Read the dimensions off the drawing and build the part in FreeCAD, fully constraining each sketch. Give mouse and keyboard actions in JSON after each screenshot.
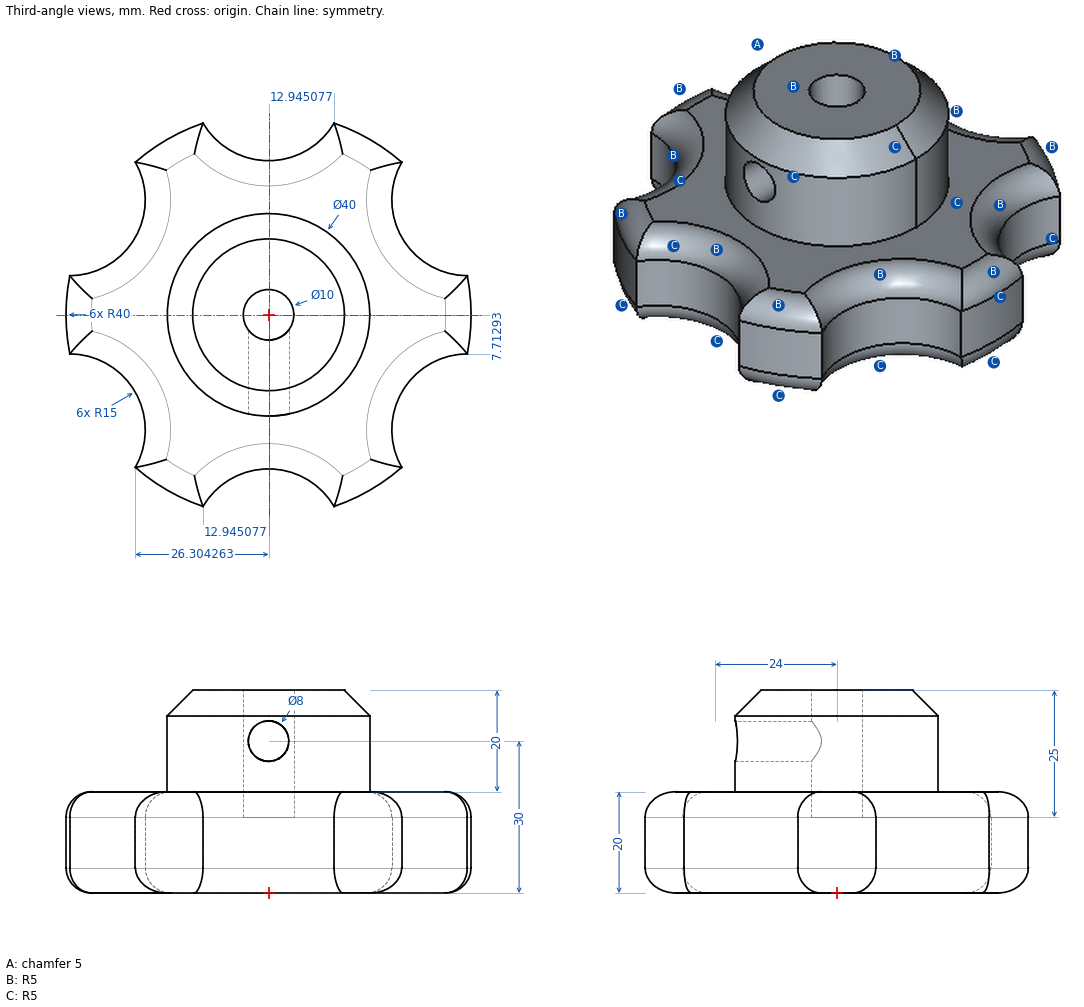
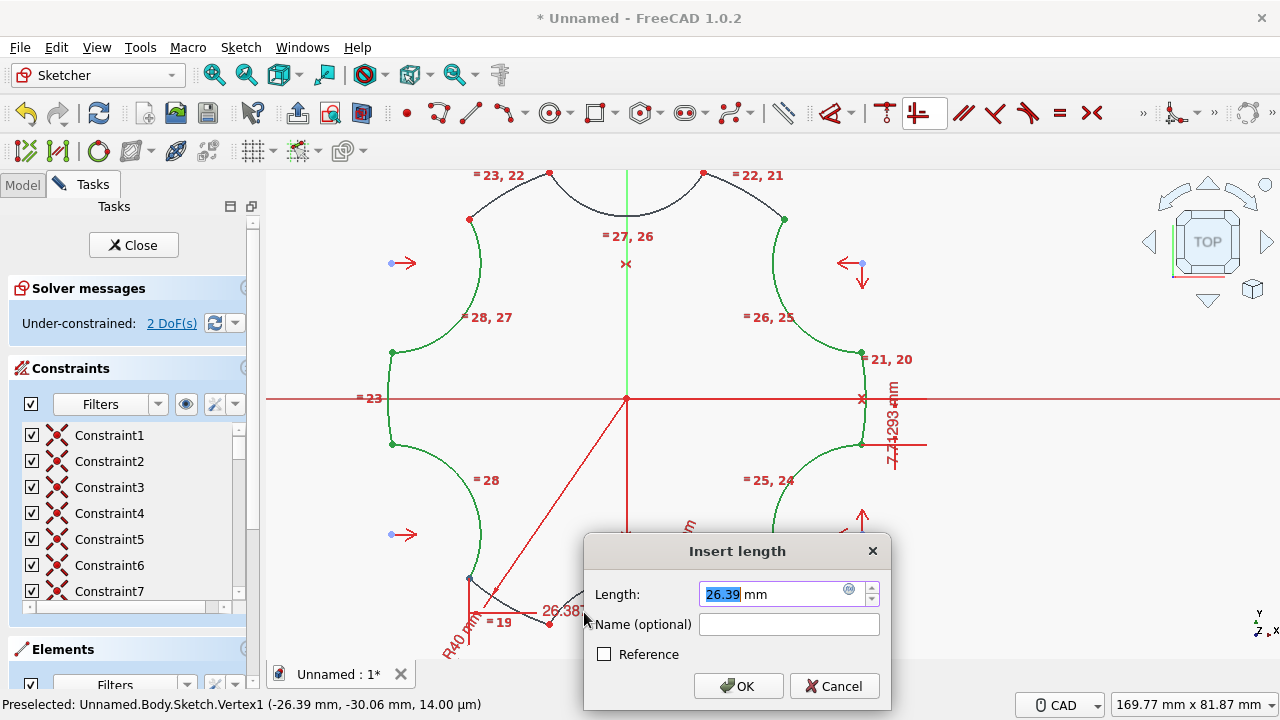
{"action": "type", "text": "26.304263"}
{"action": "key", "text": "Return"}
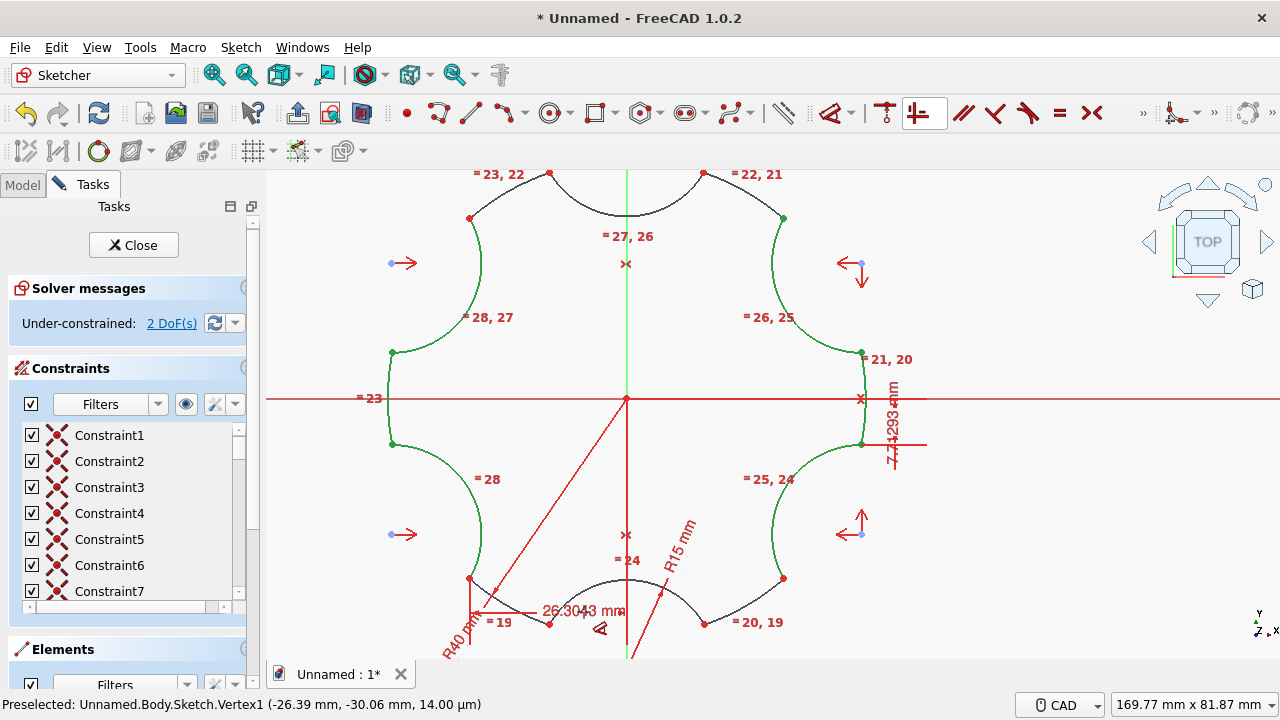
{"action": "left_click", "coordinate": [549, 625]}
{"action": "left_click", "coordinate": [588, 365]}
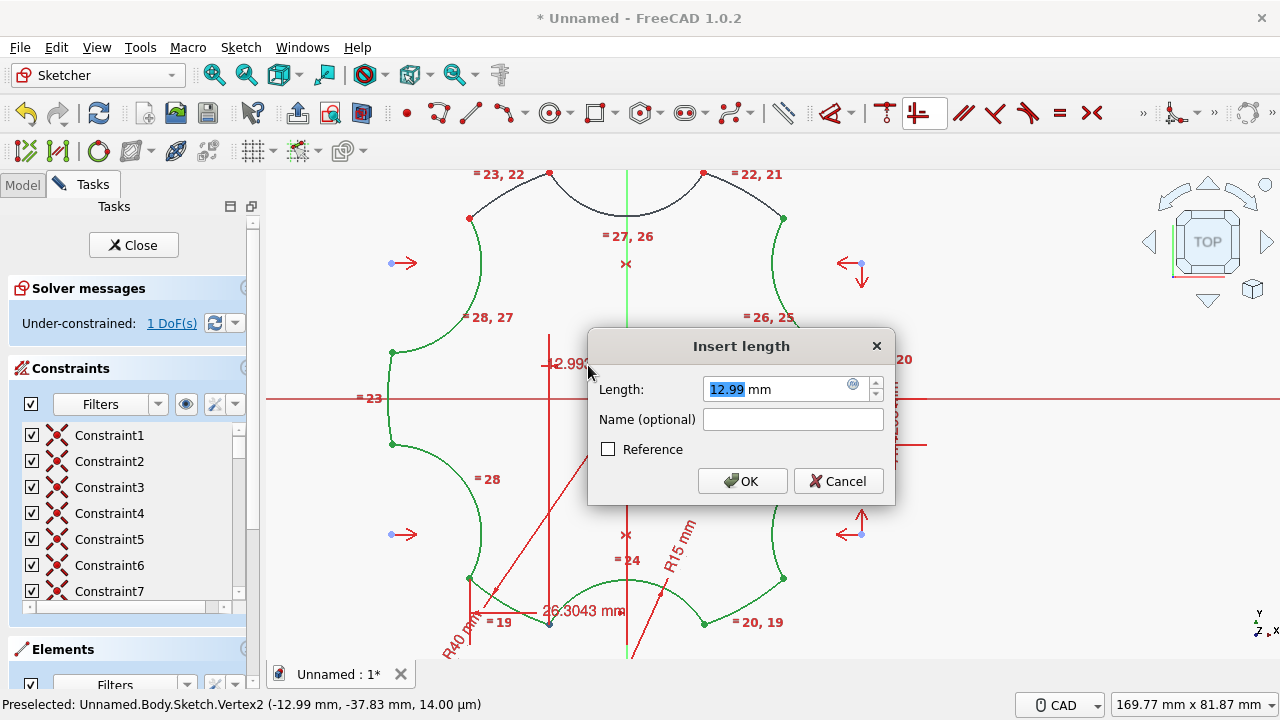
{"action": "type", "text": "12.945077"}
{"action": "key", "text": "Return"}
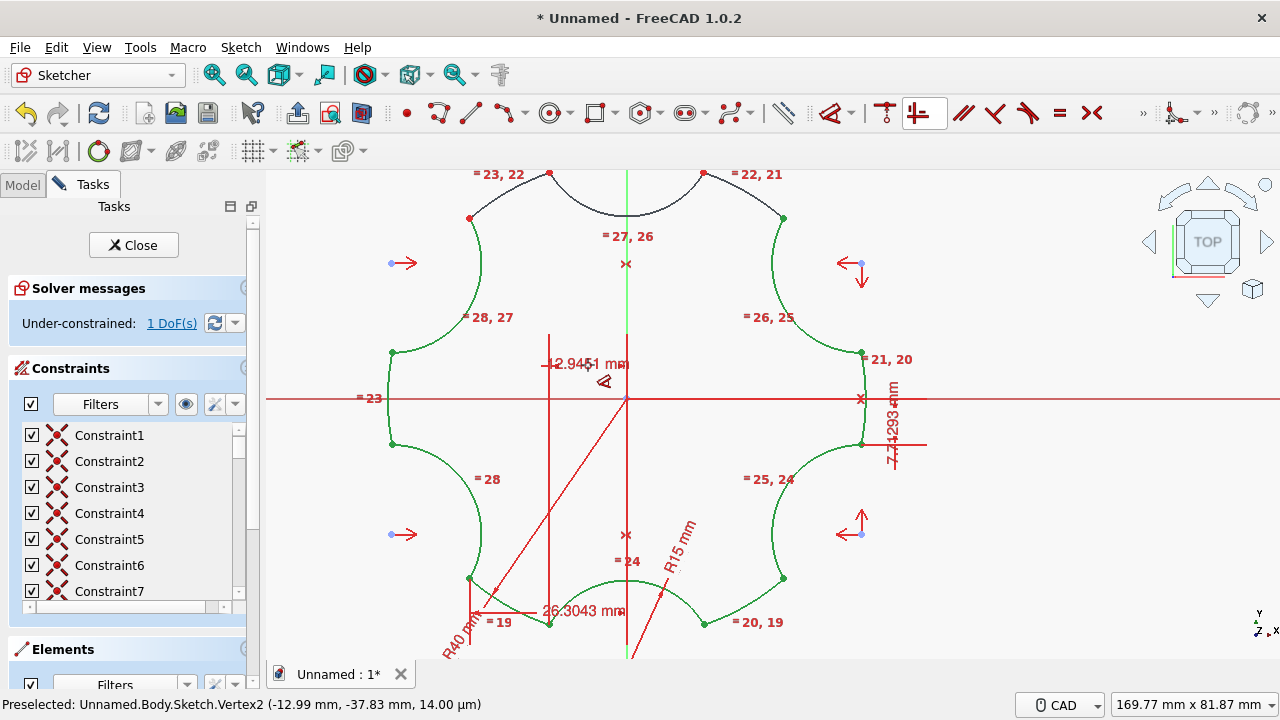
{"action": "scroll", "coordinate": [863, 446], "scroll_direction": "down", "scroll_amount": 2}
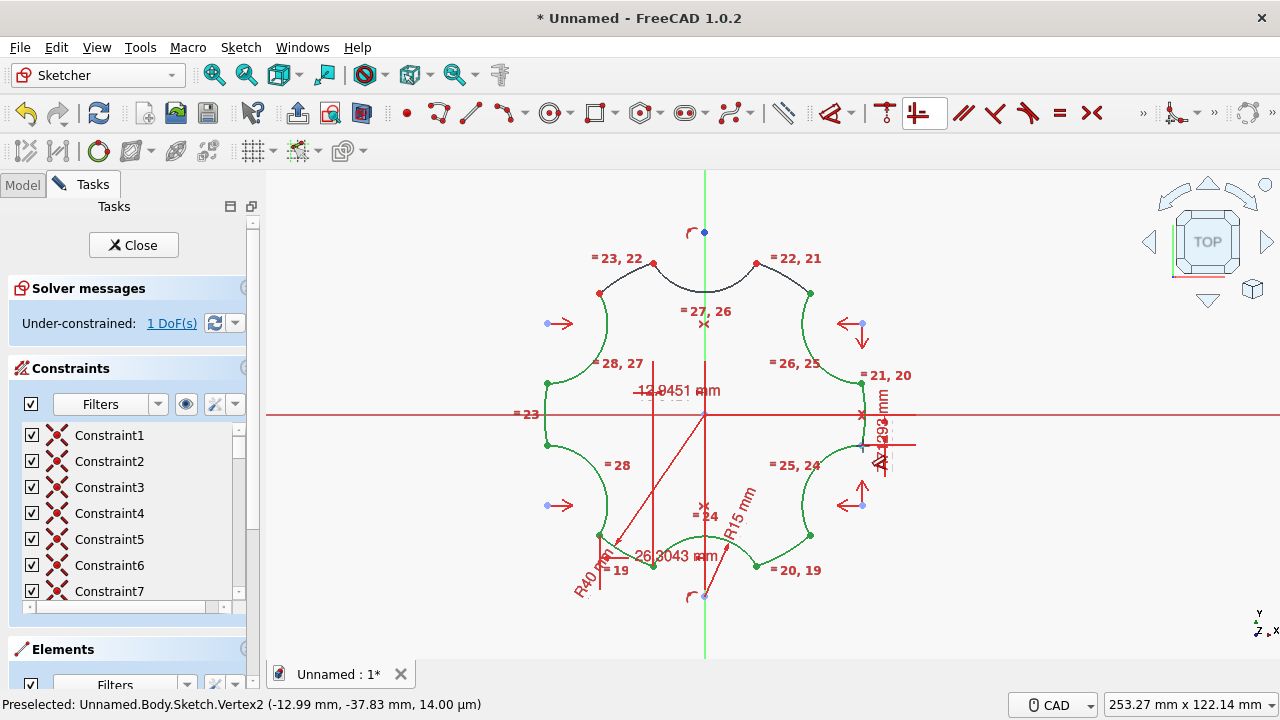
{"action": "left_click", "coordinate": [756, 263]}
{"action": "left_click", "coordinate": [731, 229]}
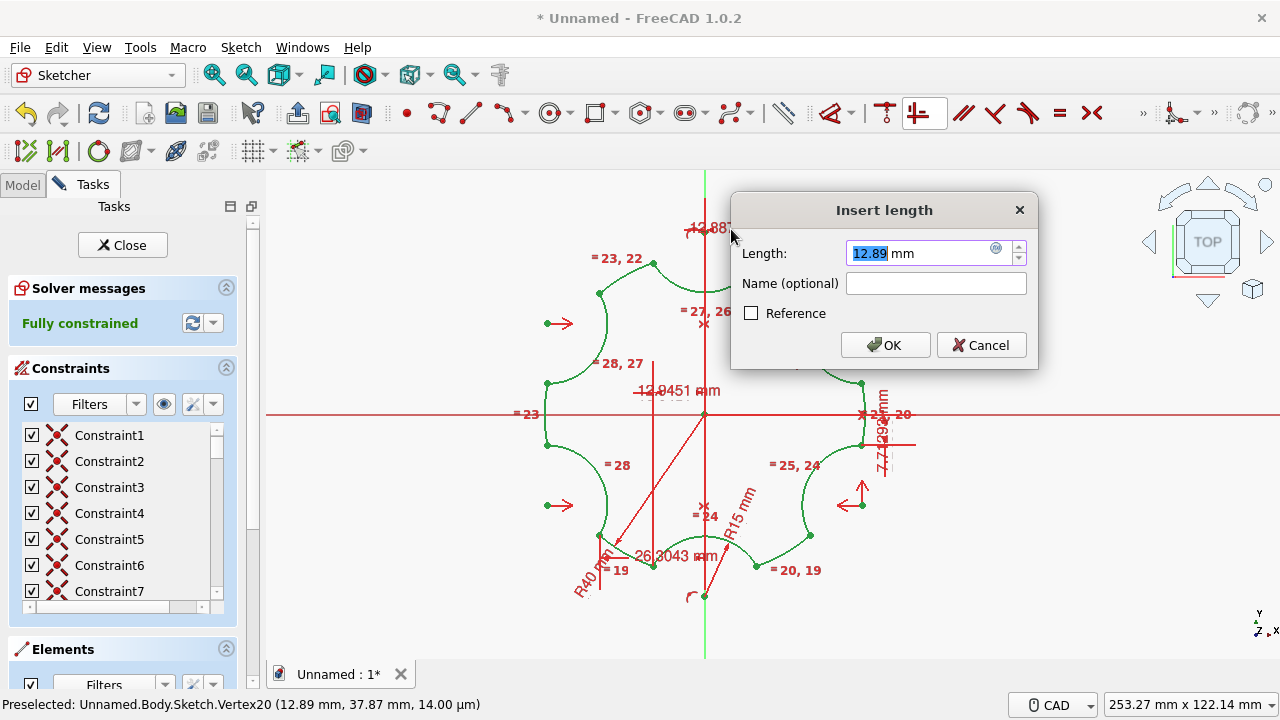
{"action": "type", "text": "12.945077"}
{"action": "key", "text": "Return"}
{"action": "key", "text": "Escape"}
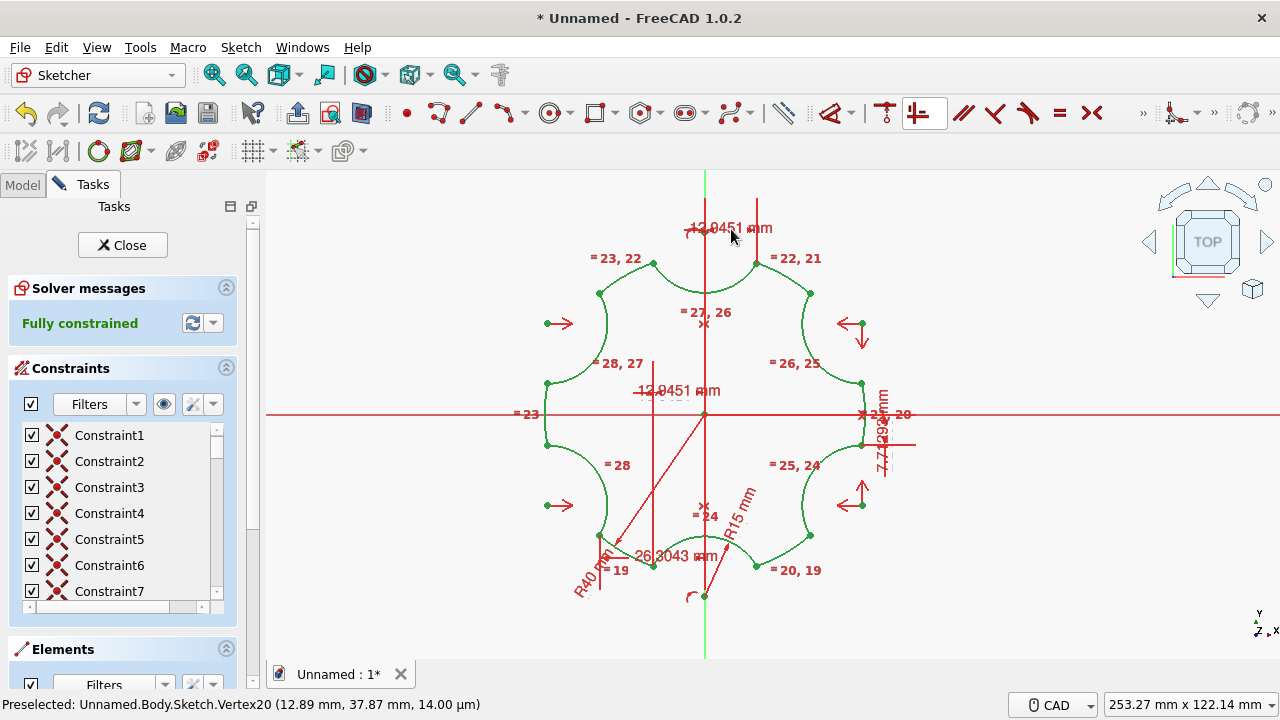
{"action": "left_click", "coordinate": [123, 245]}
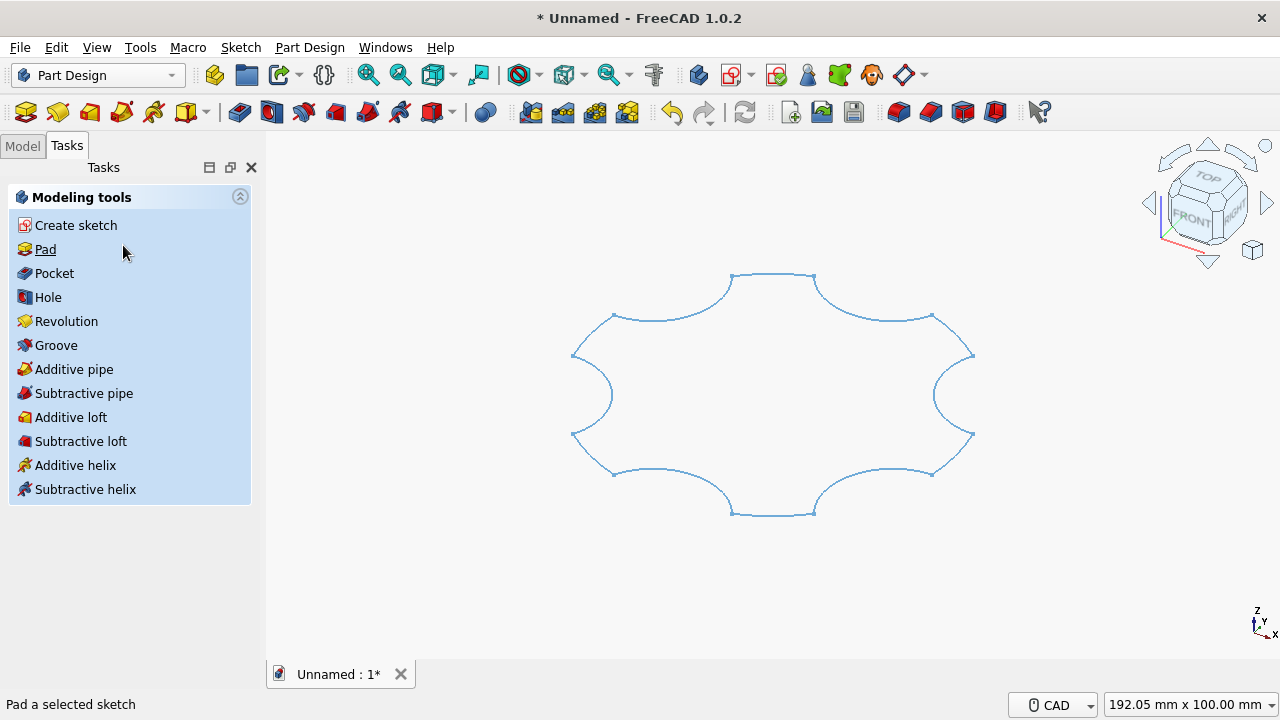
{"action": "left_click", "coordinate": [26, 112]}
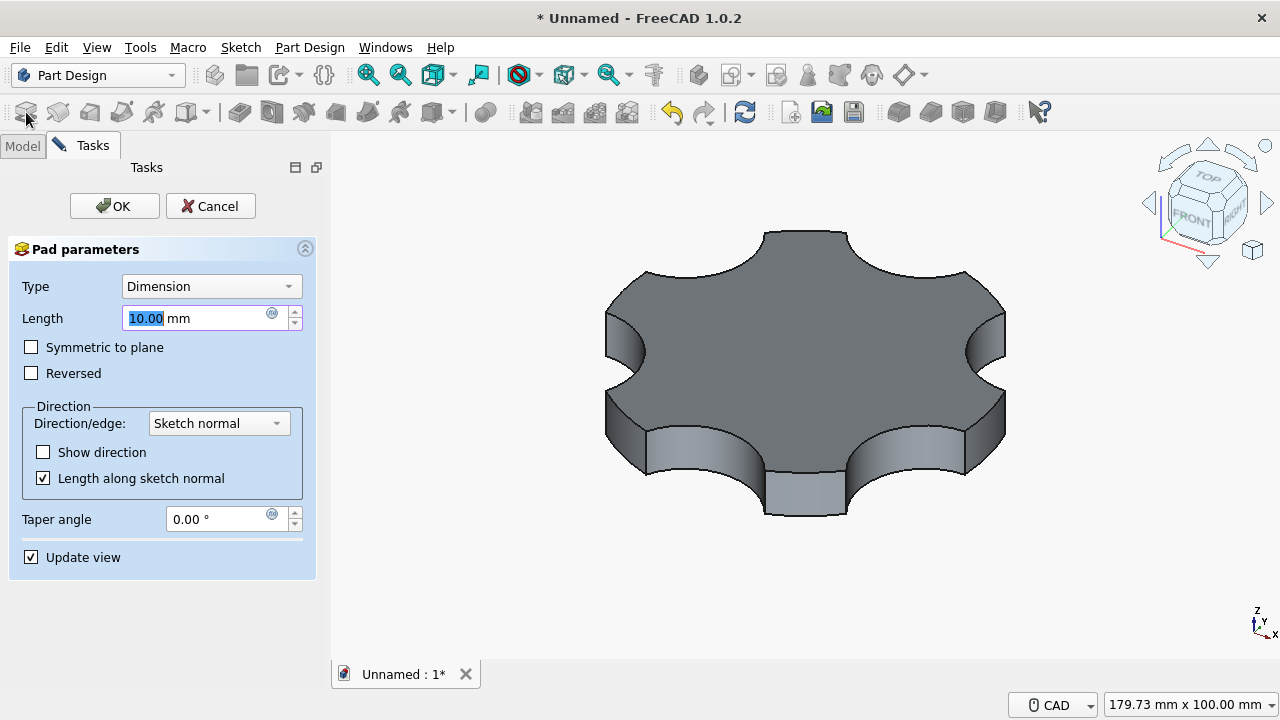
{"action": "type", "text": "20"}
{"action": "key", "text": "Tab"}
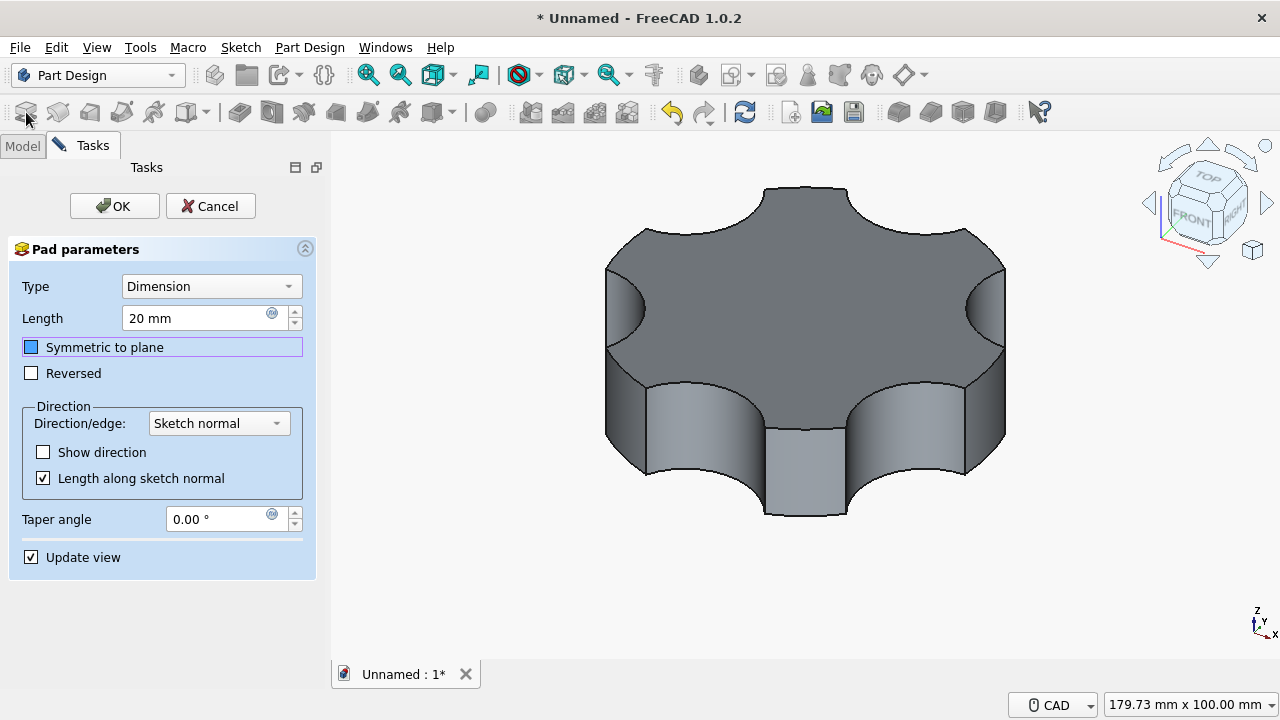
{"action": "left_click", "coordinate": [115, 206]}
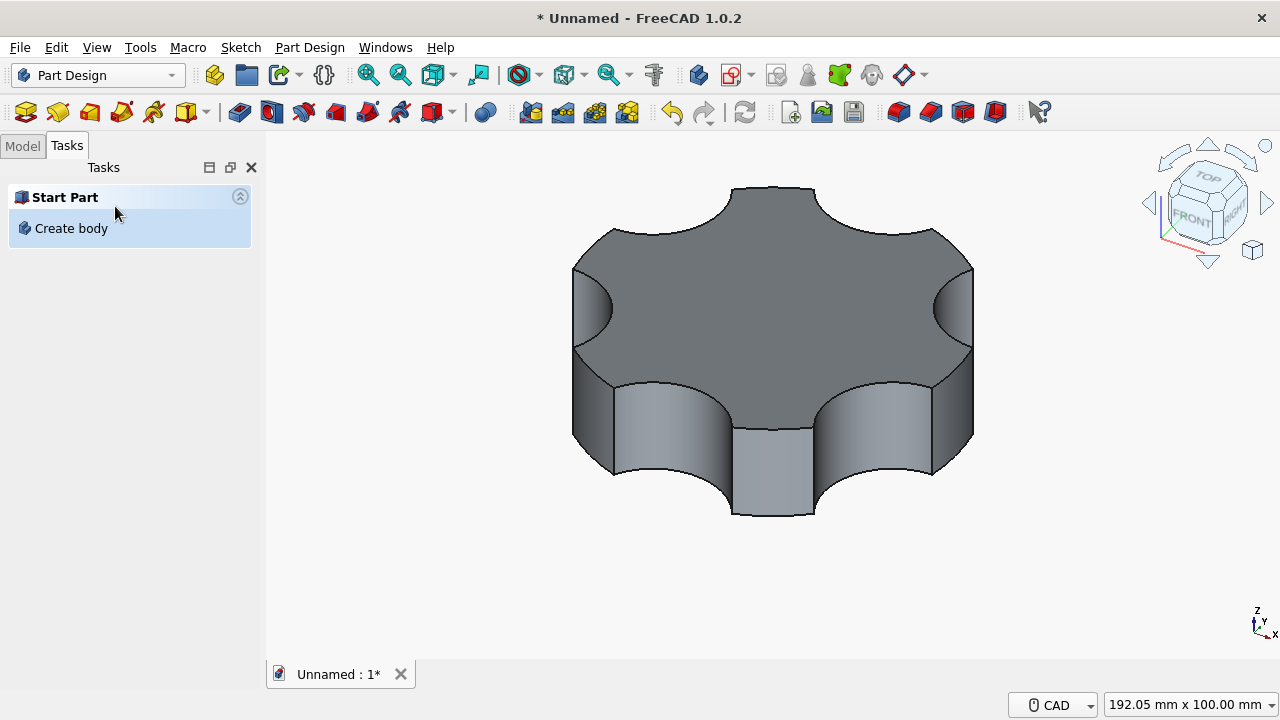
{"action": "left_click", "coordinate": [773, 307]}